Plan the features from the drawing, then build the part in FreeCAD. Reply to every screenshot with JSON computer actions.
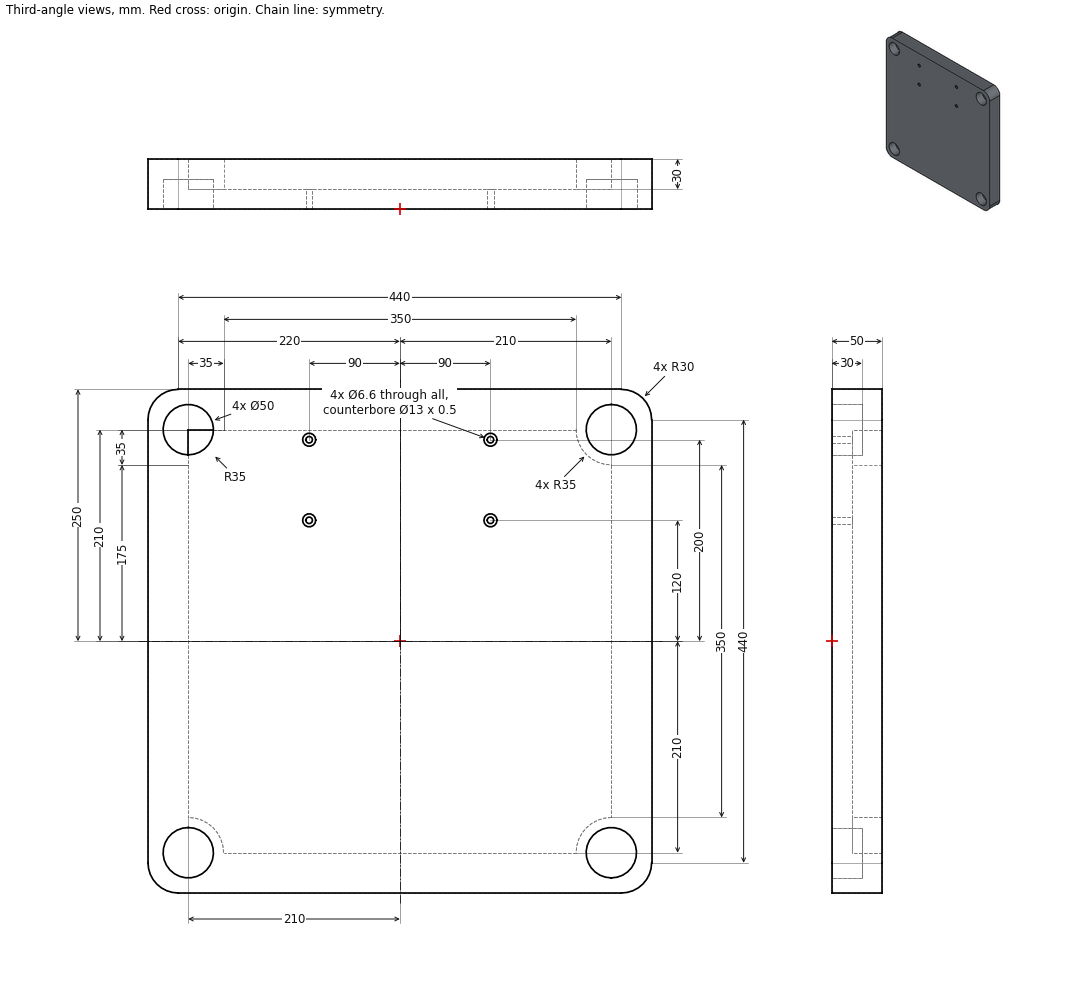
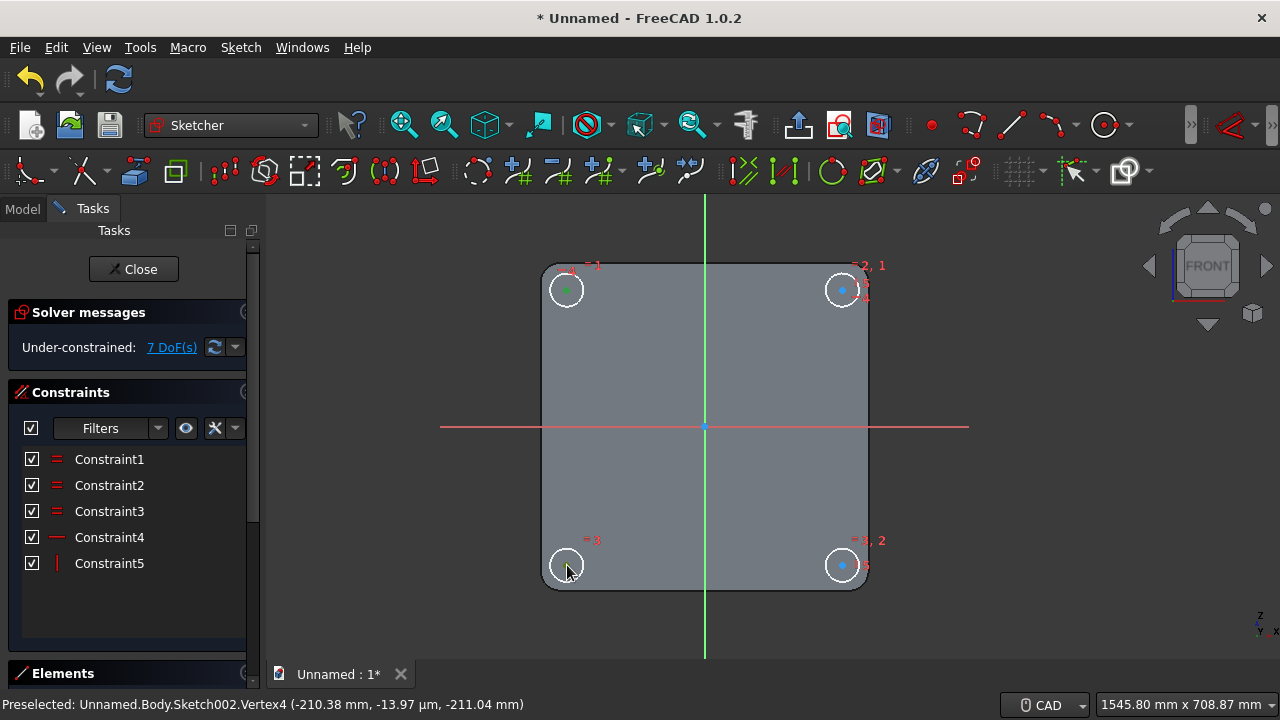
{"action": "key", "text": "v"}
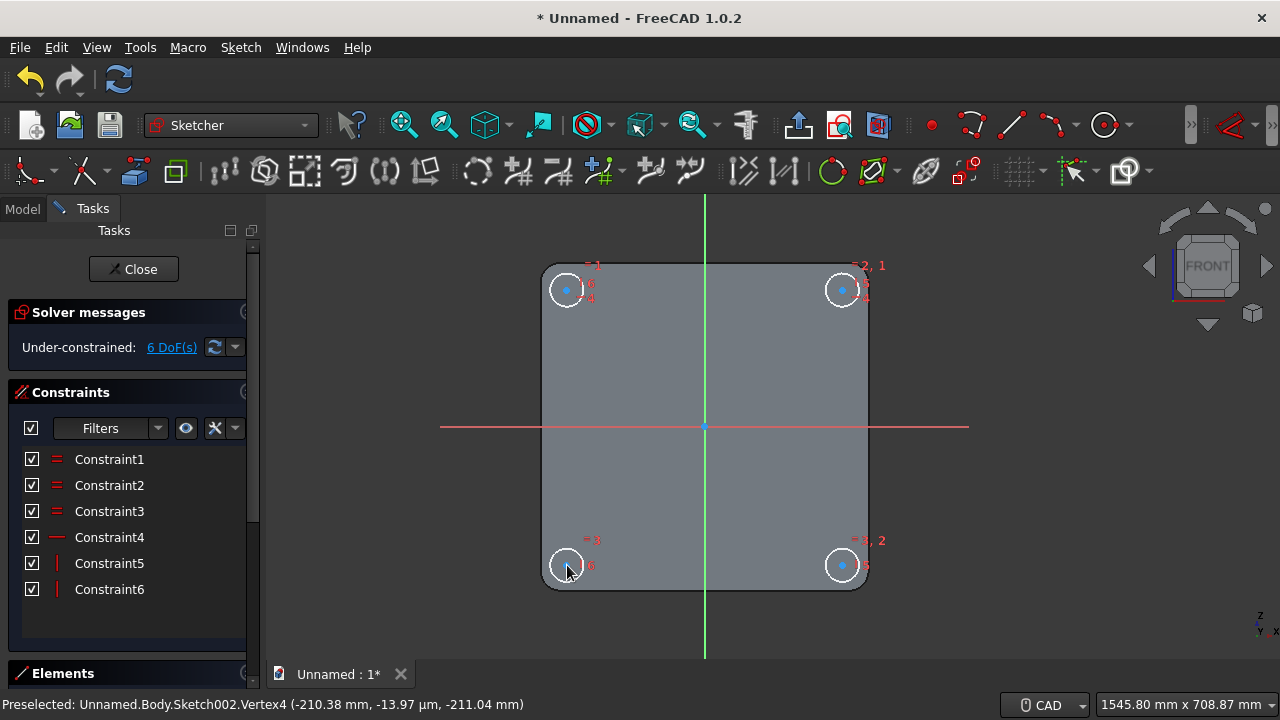
{"action": "left_click", "coordinate": [842, 565]}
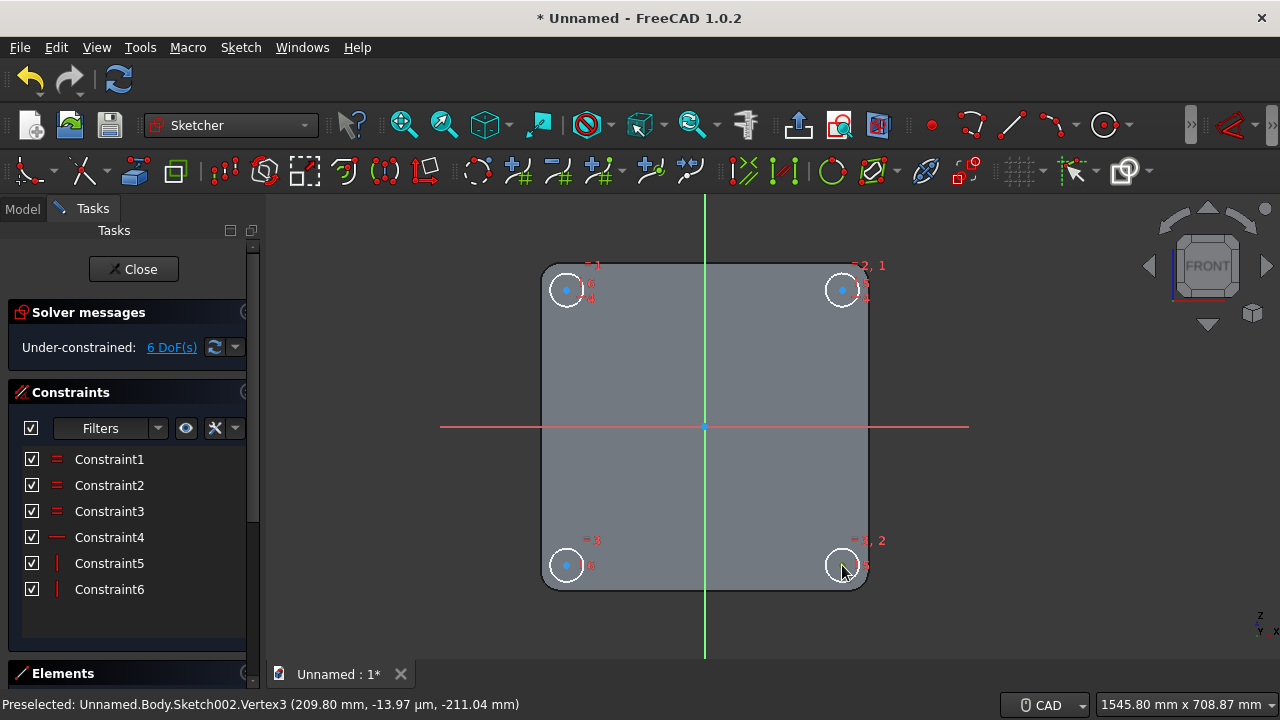
{"action": "left_click", "coordinate": [567, 565]}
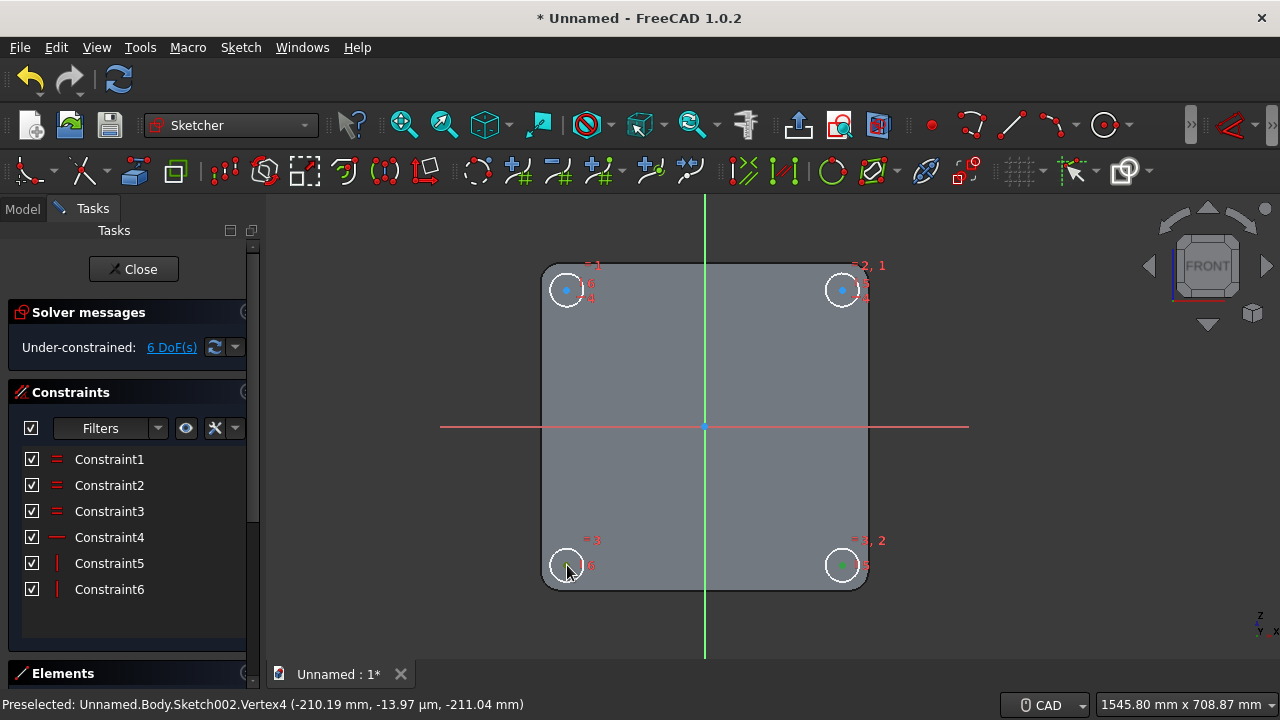
{"action": "key", "text": "h"}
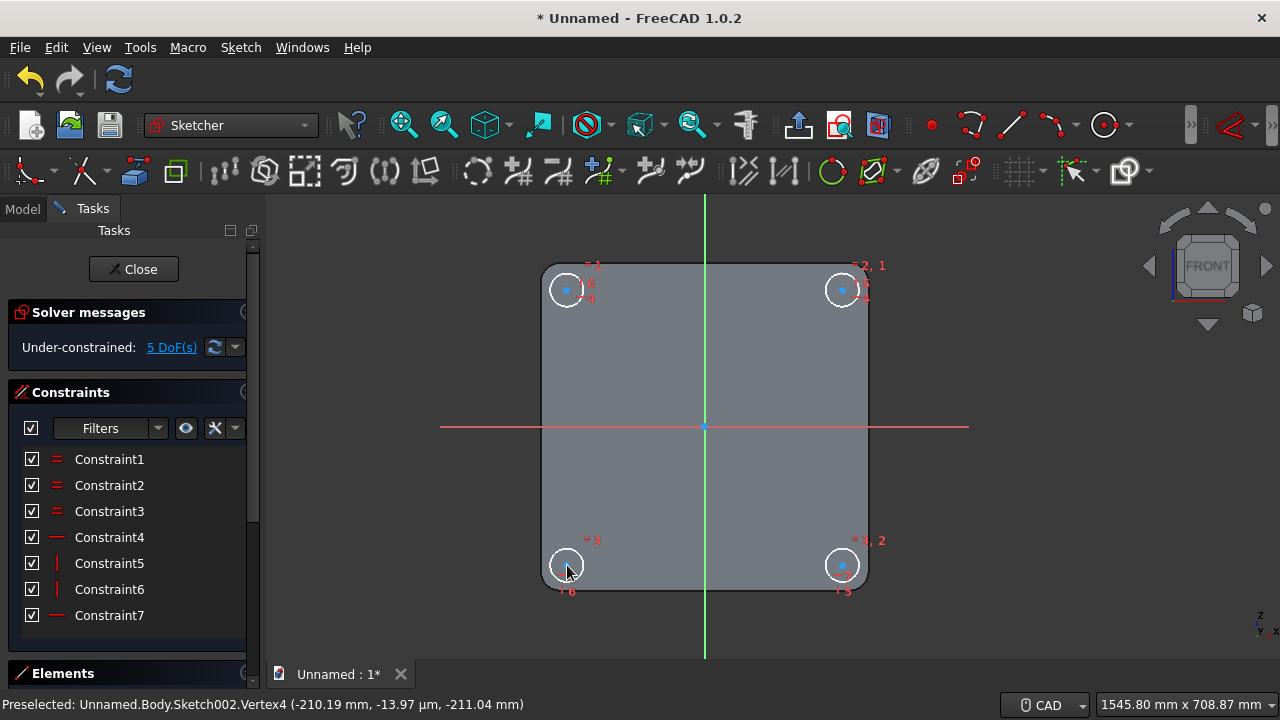
{"action": "key", "text": "d"}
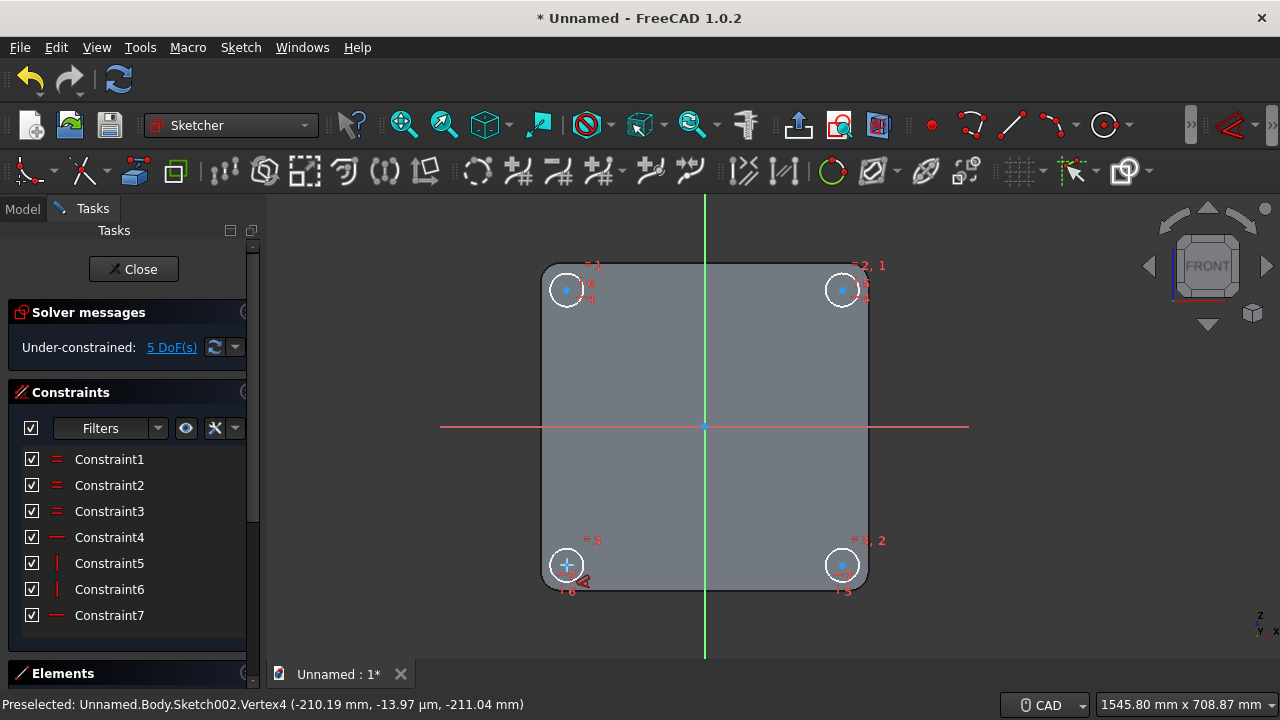
{"action": "left_click", "coordinate": [579, 278]}
{"action": "left_click", "coordinate": [602, 255]}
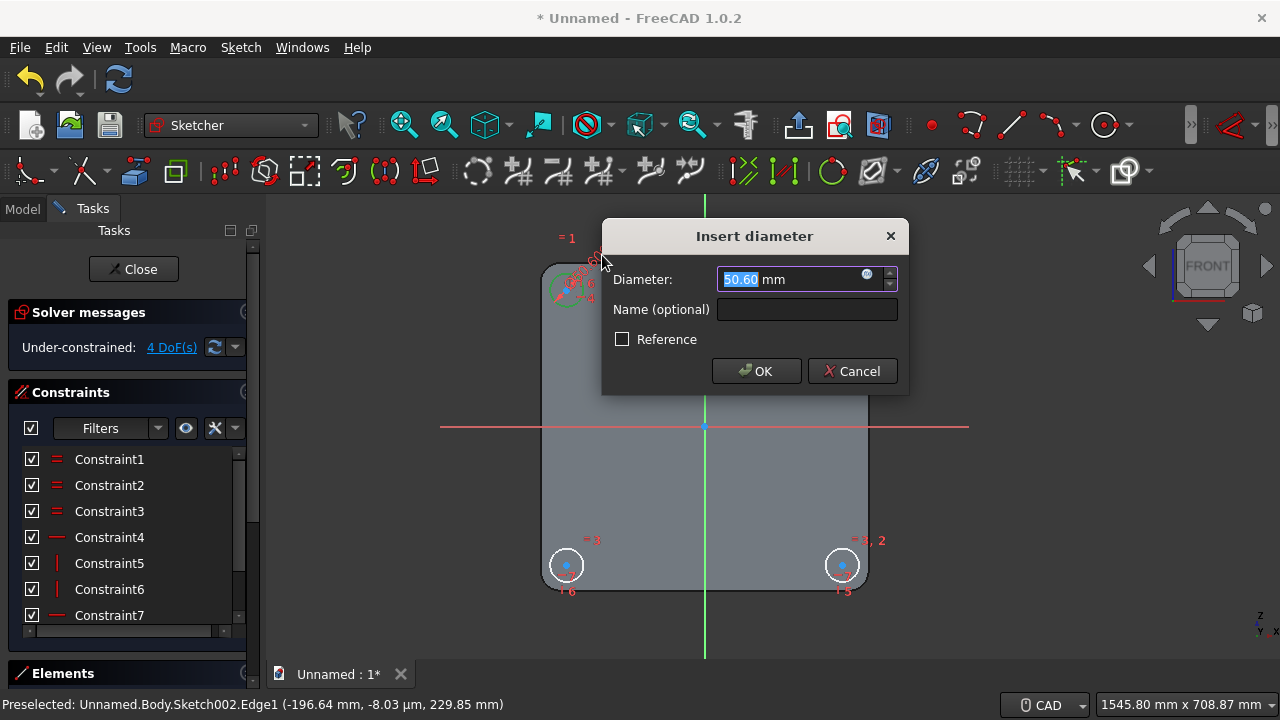
{"action": "type", "text": "50"}
{"action": "key", "text": "Return"}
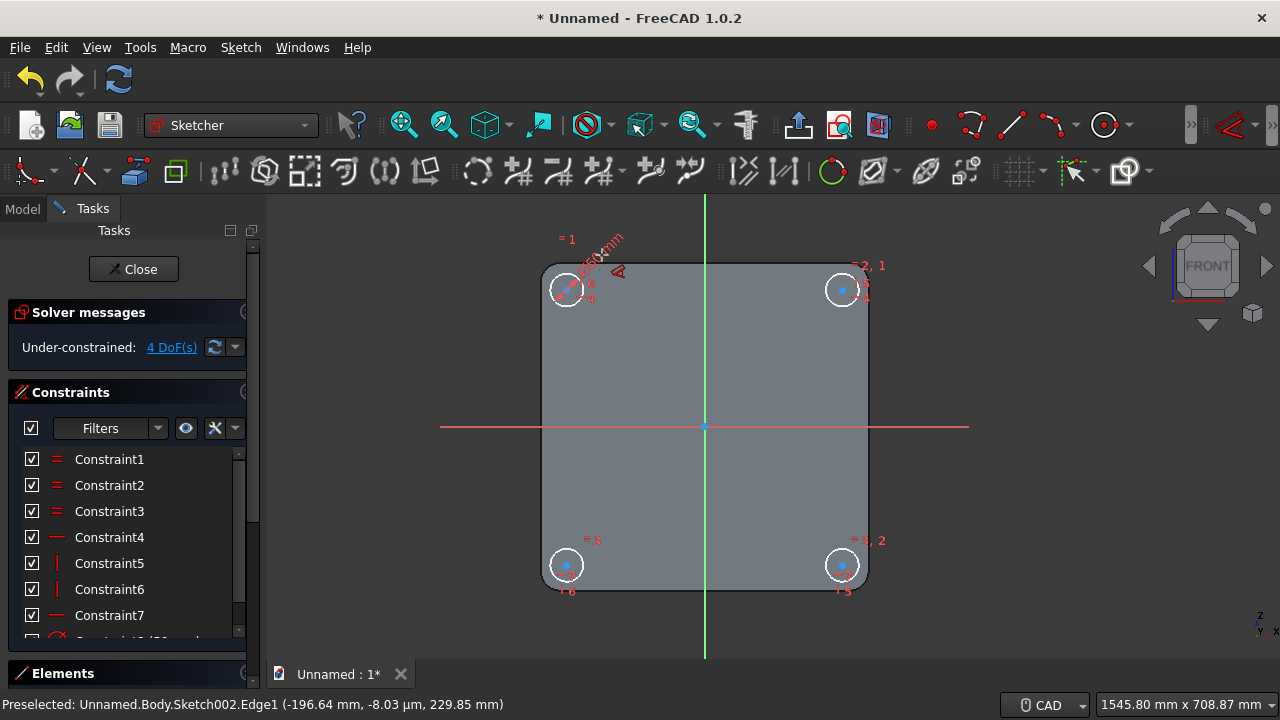
{"action": "left_click", "coordinate": [567, 290]}
{"action": "left_click", "coordinate": [684, 256]}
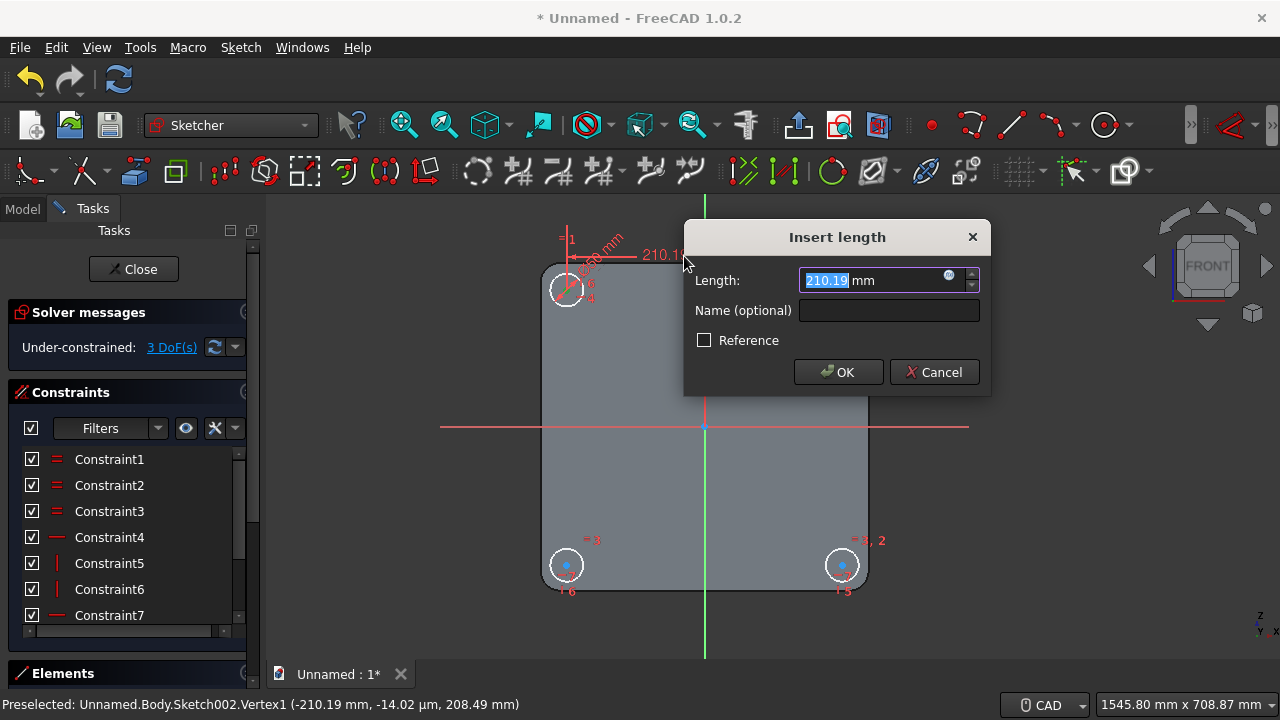
{"action": "type", "text": "210"}
{"action": "key", "text": "Return"}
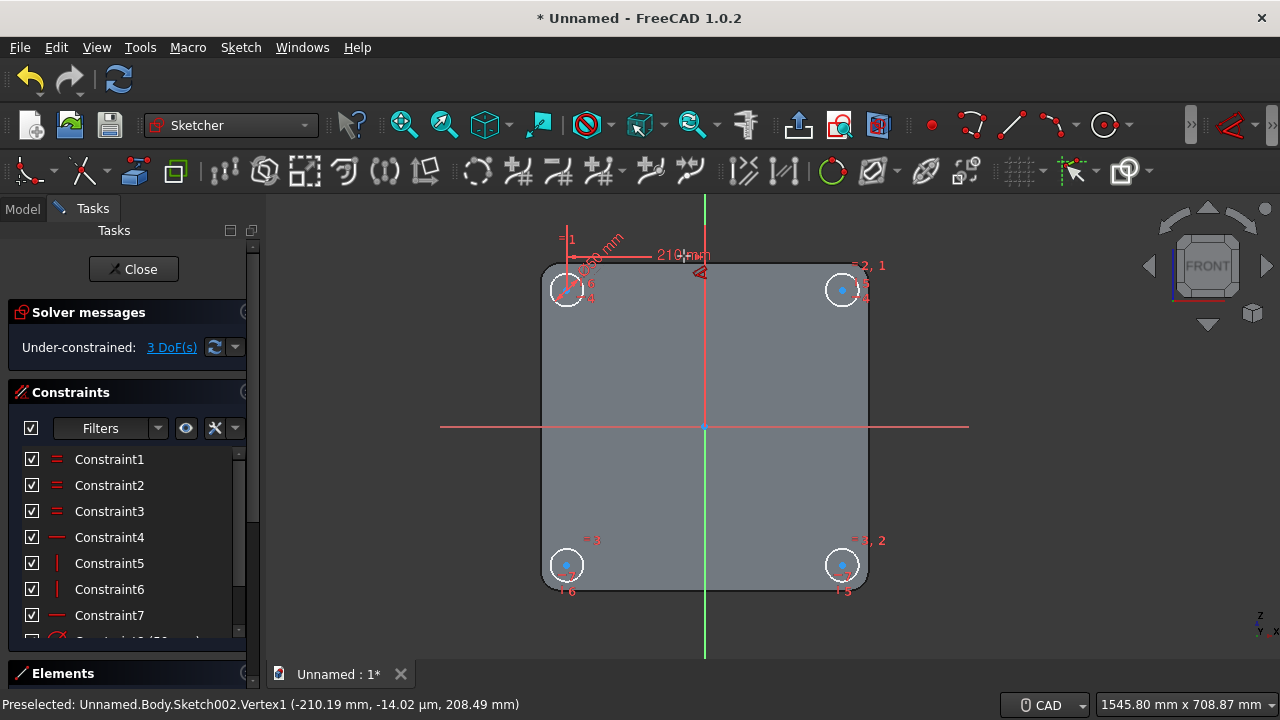
{"action": "left_click", "coordinate": [567, 290]}
{"action": "left_click", "coordinate": [533, 358]}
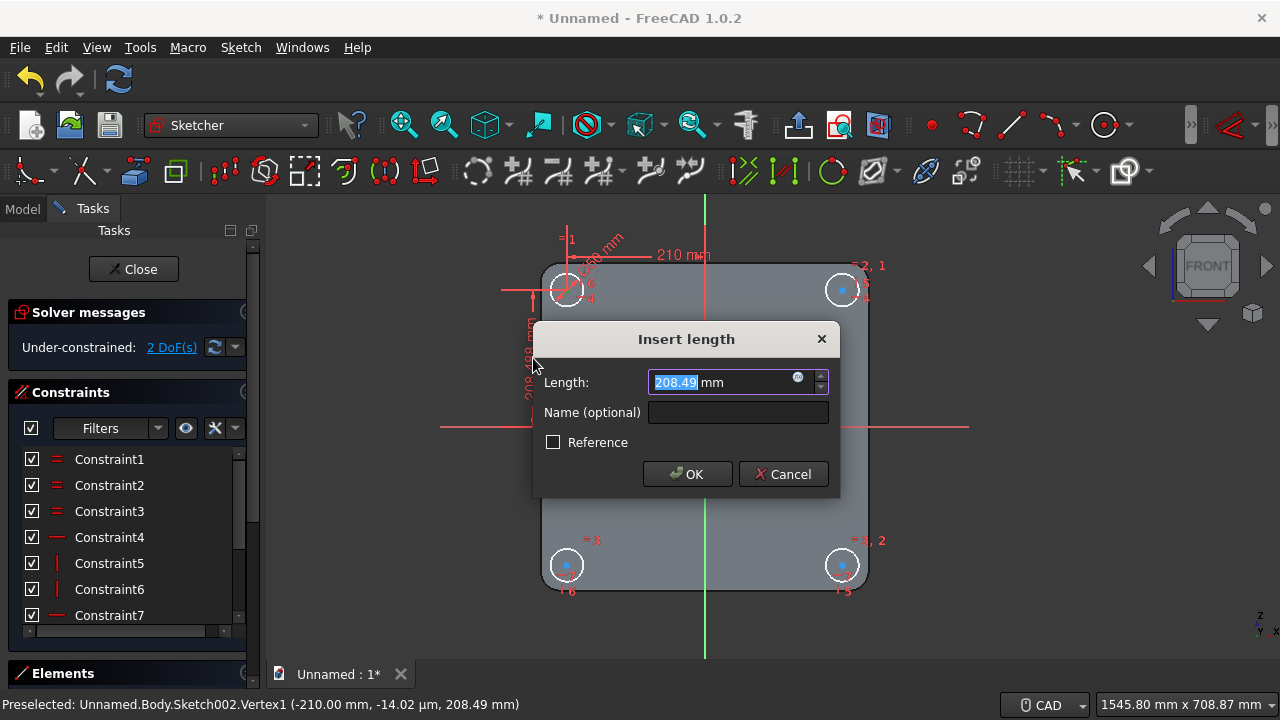
{"action": "type", "text": "210"}
{"action": "key", "text": "Return"}